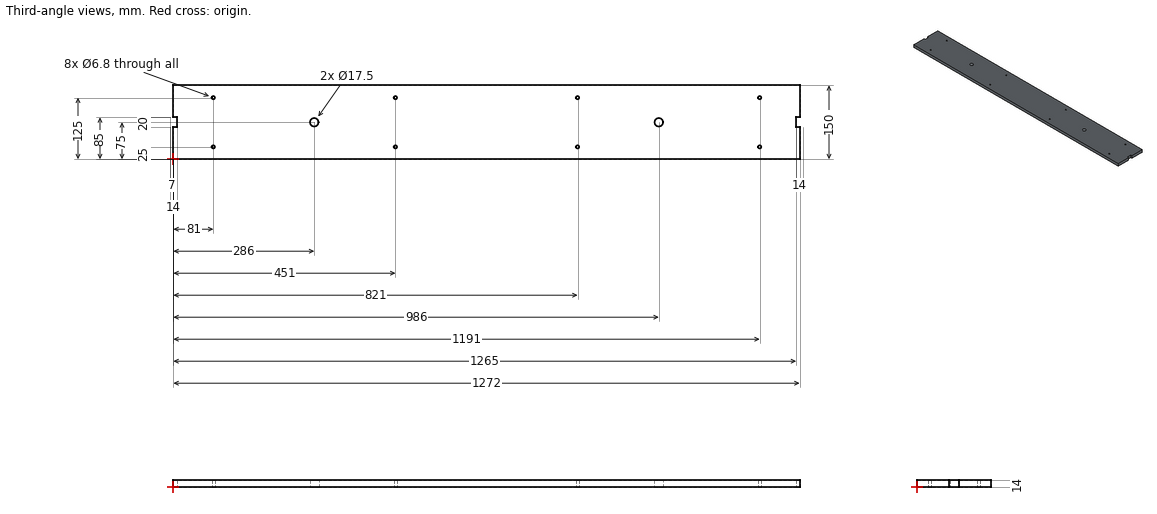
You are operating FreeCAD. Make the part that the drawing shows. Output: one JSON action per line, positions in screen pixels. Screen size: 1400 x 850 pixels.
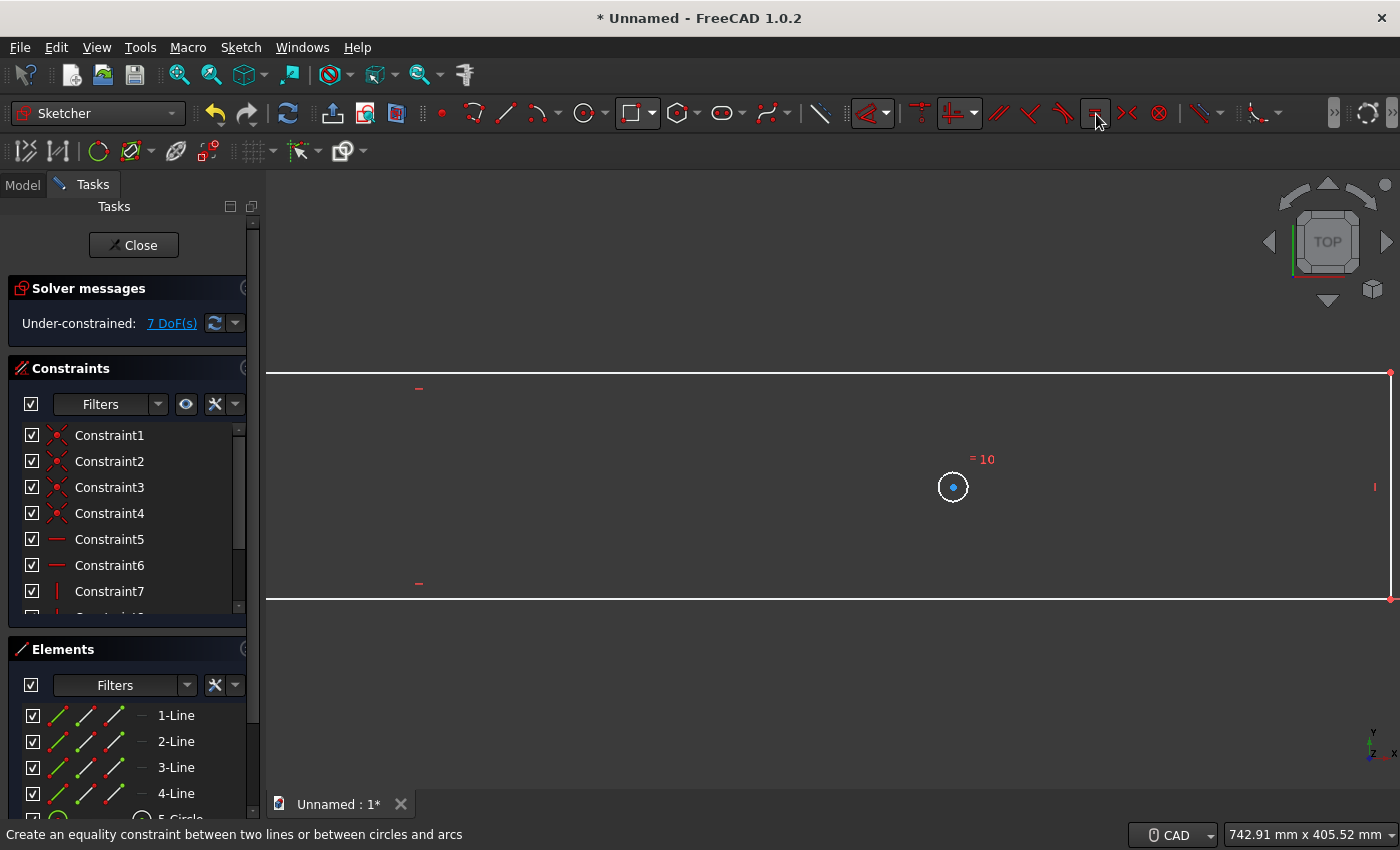
{"action": "scroll", "coordinate": [965, 476], "scroll_direction": "down", "scroll_amount": 5}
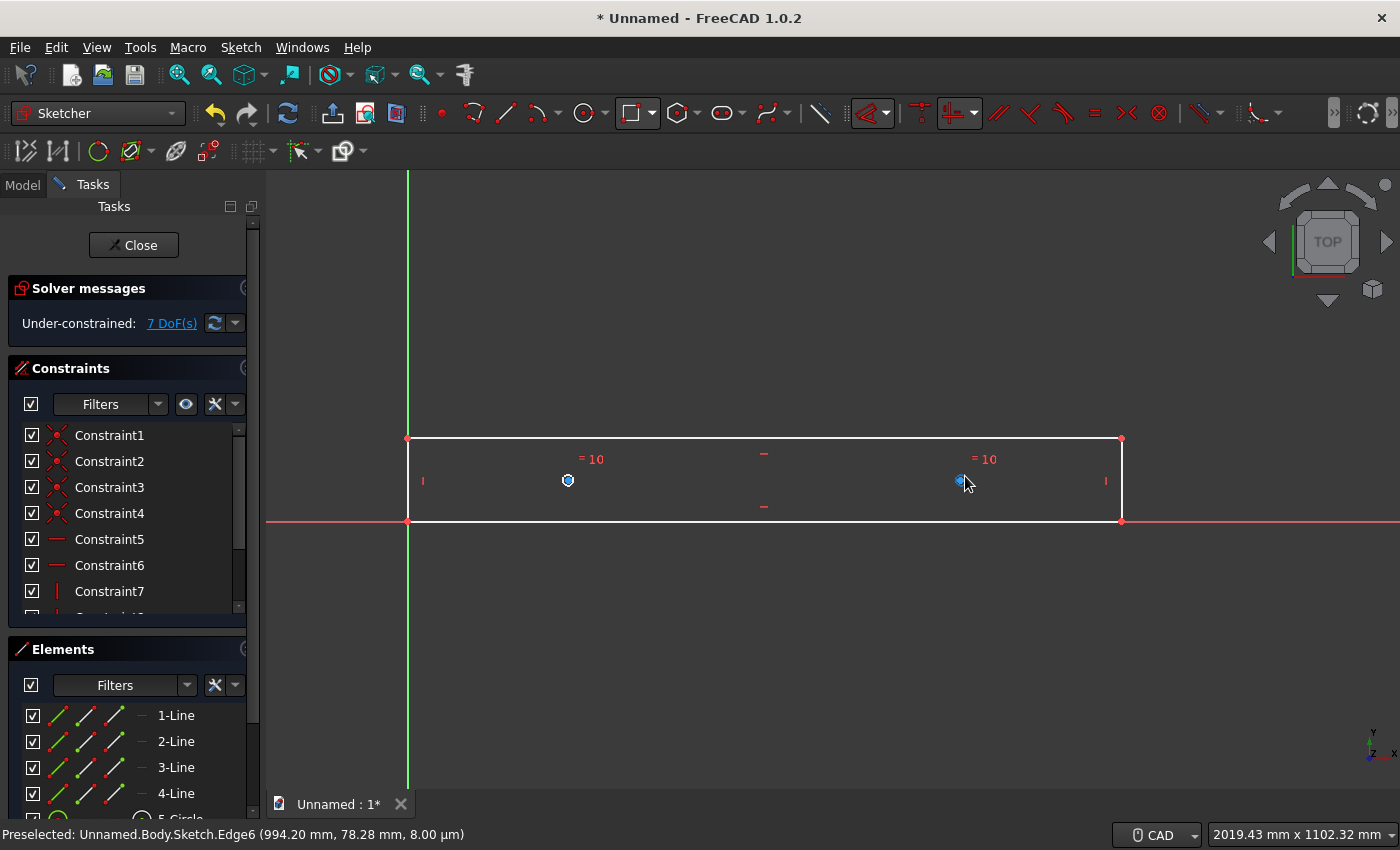
{"action": "left_click", "coordinate": [568, 480]}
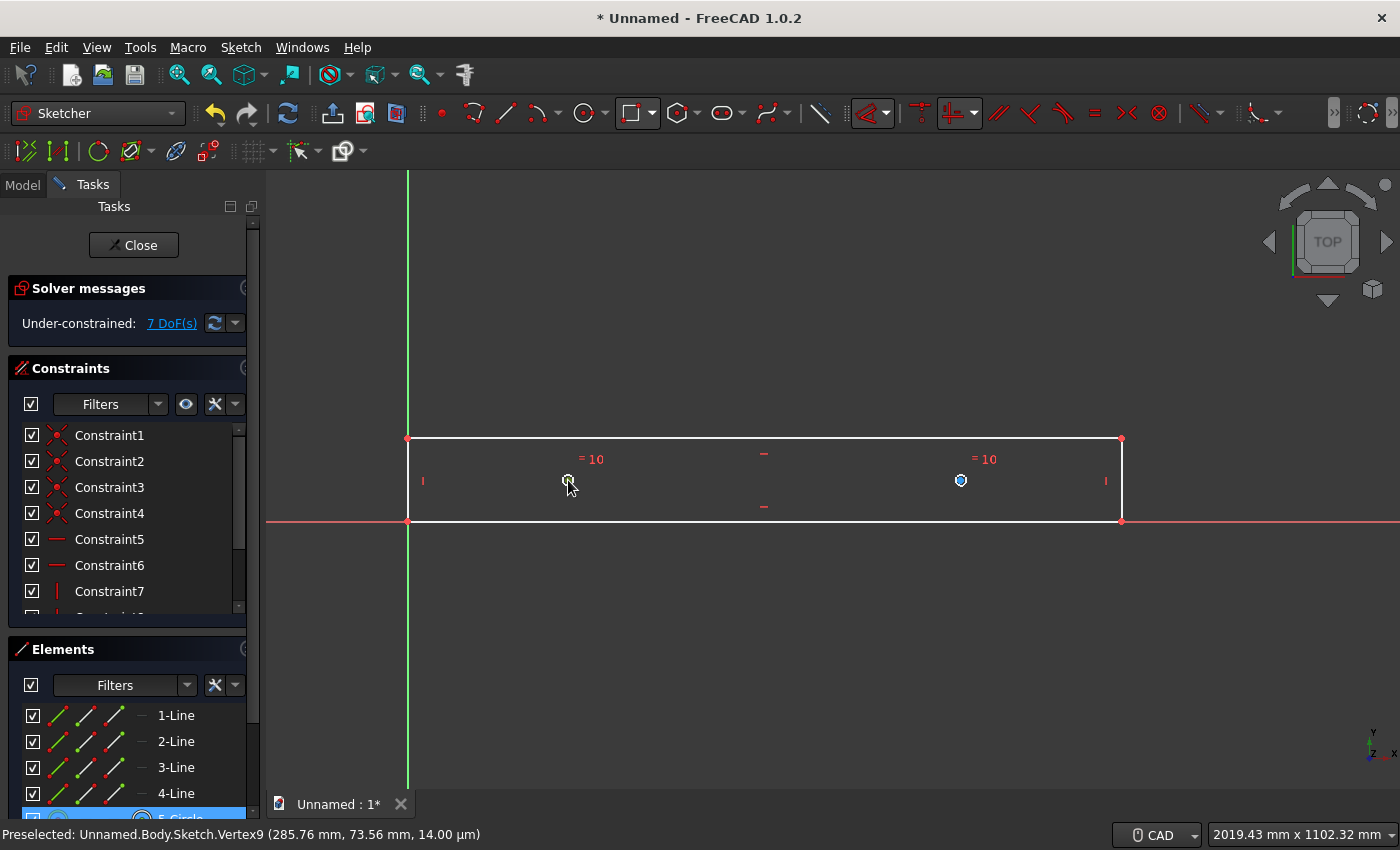
{"action": "left_click", "coordinate": [961, 480]}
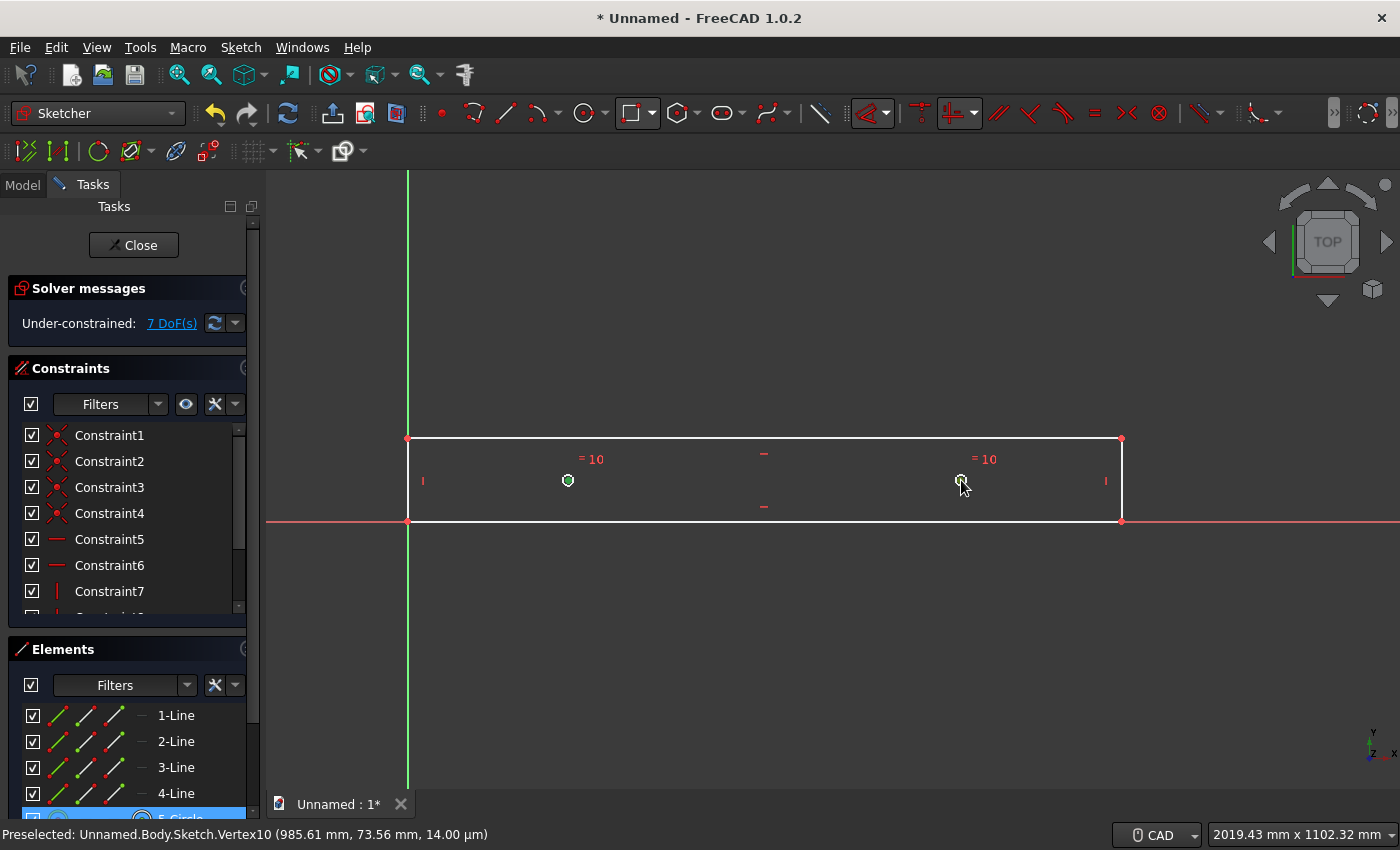
{"action": "left_click", "coordinate": [976, 114]}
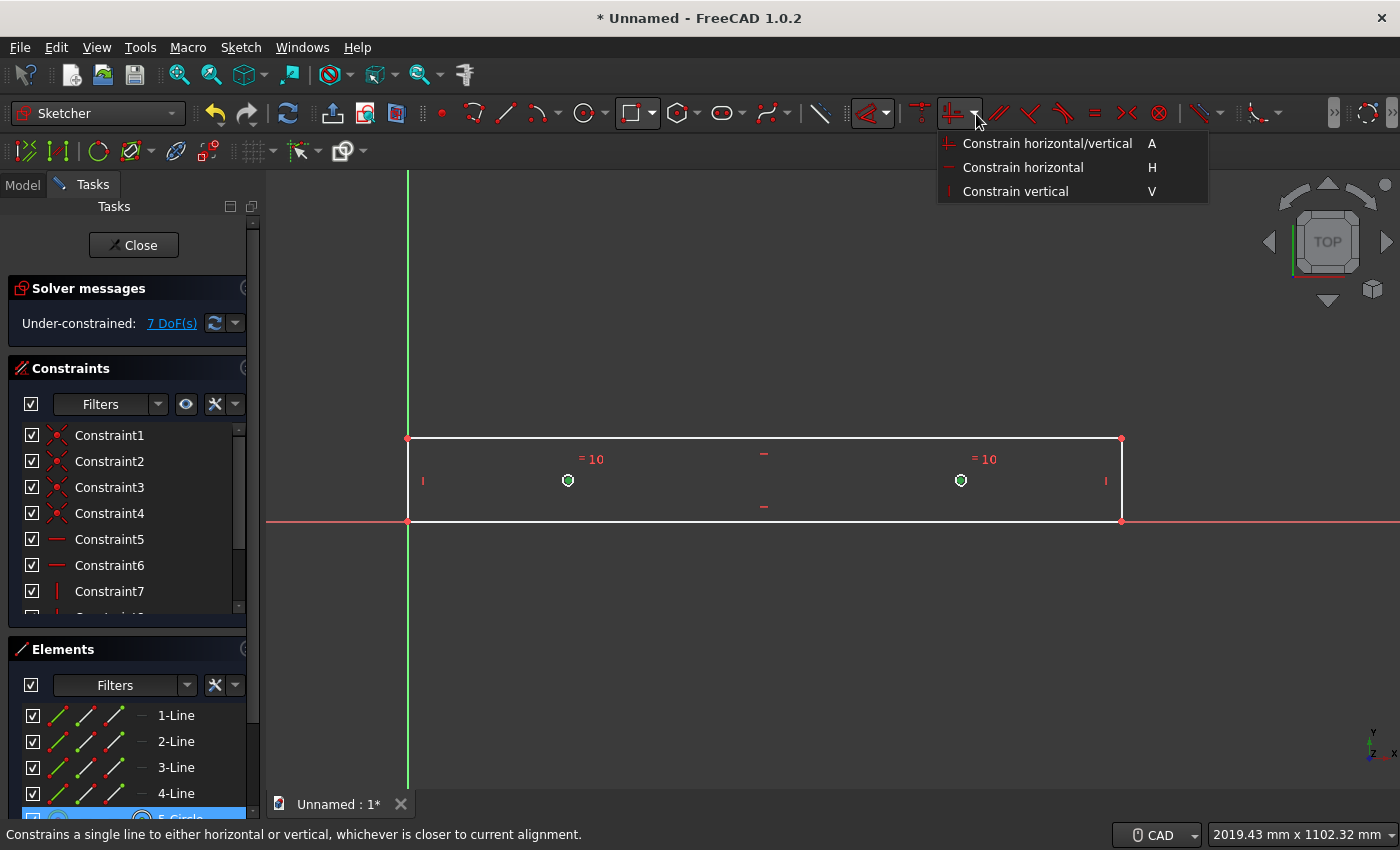
{"action": "left_click", "coordinate": [1073, 167]}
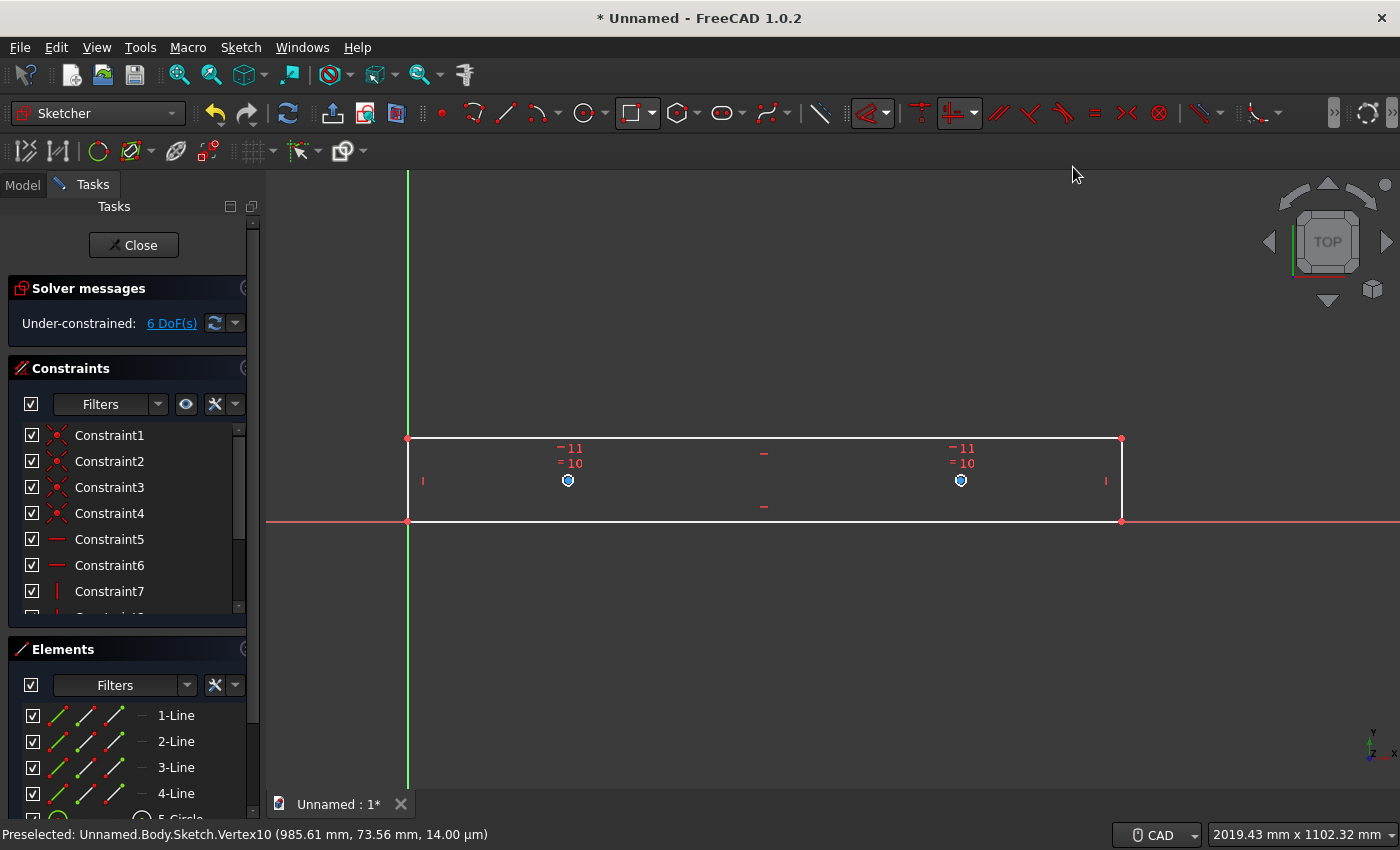
{"action": "scroll", "coordinate": [563, 480], "scroll_direction": "up", "scroll_amount": 7}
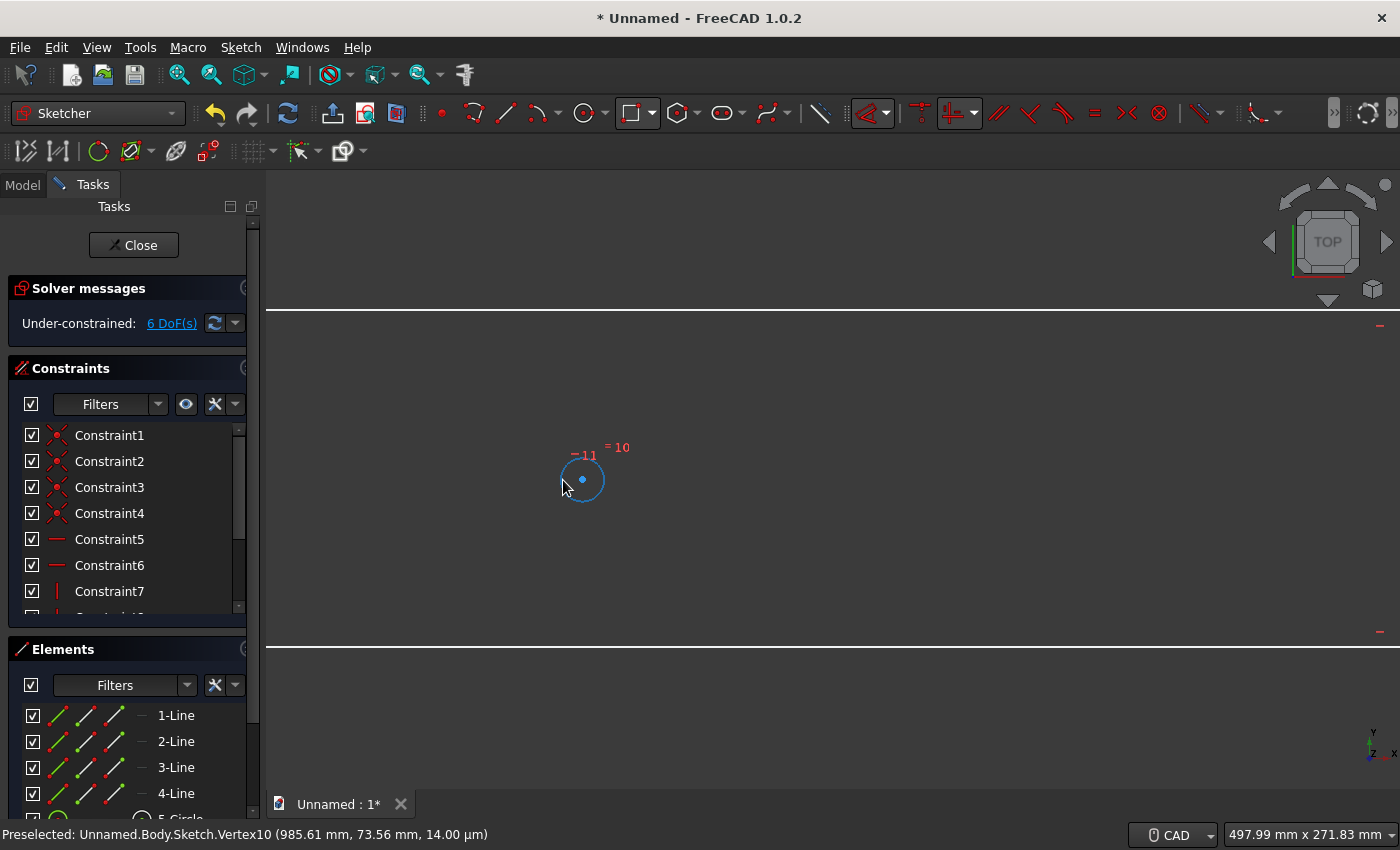
{"action": "left_click", "coordinate": [561, 479]}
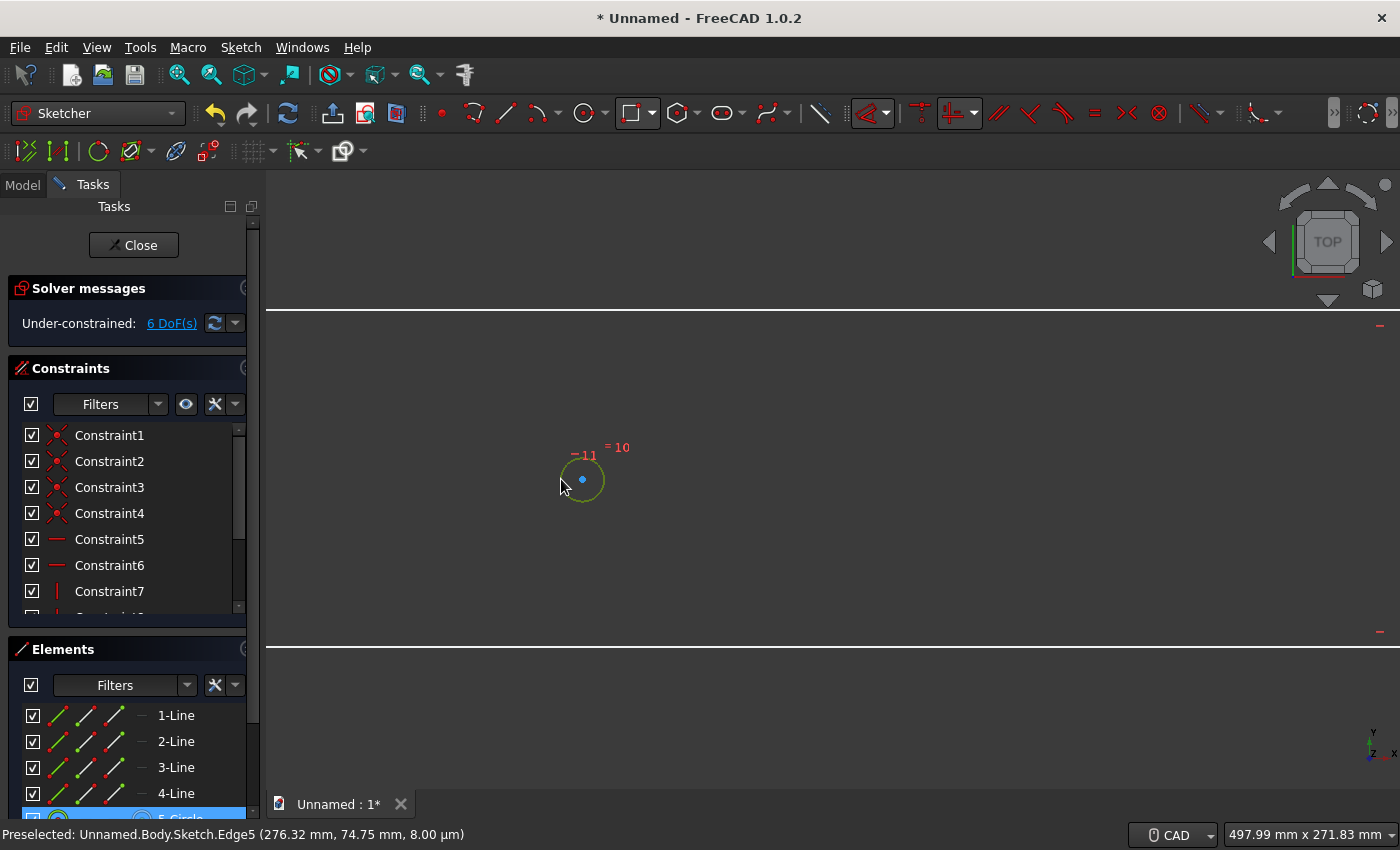
{"action": "left_click", "coordinate": [888, 114]}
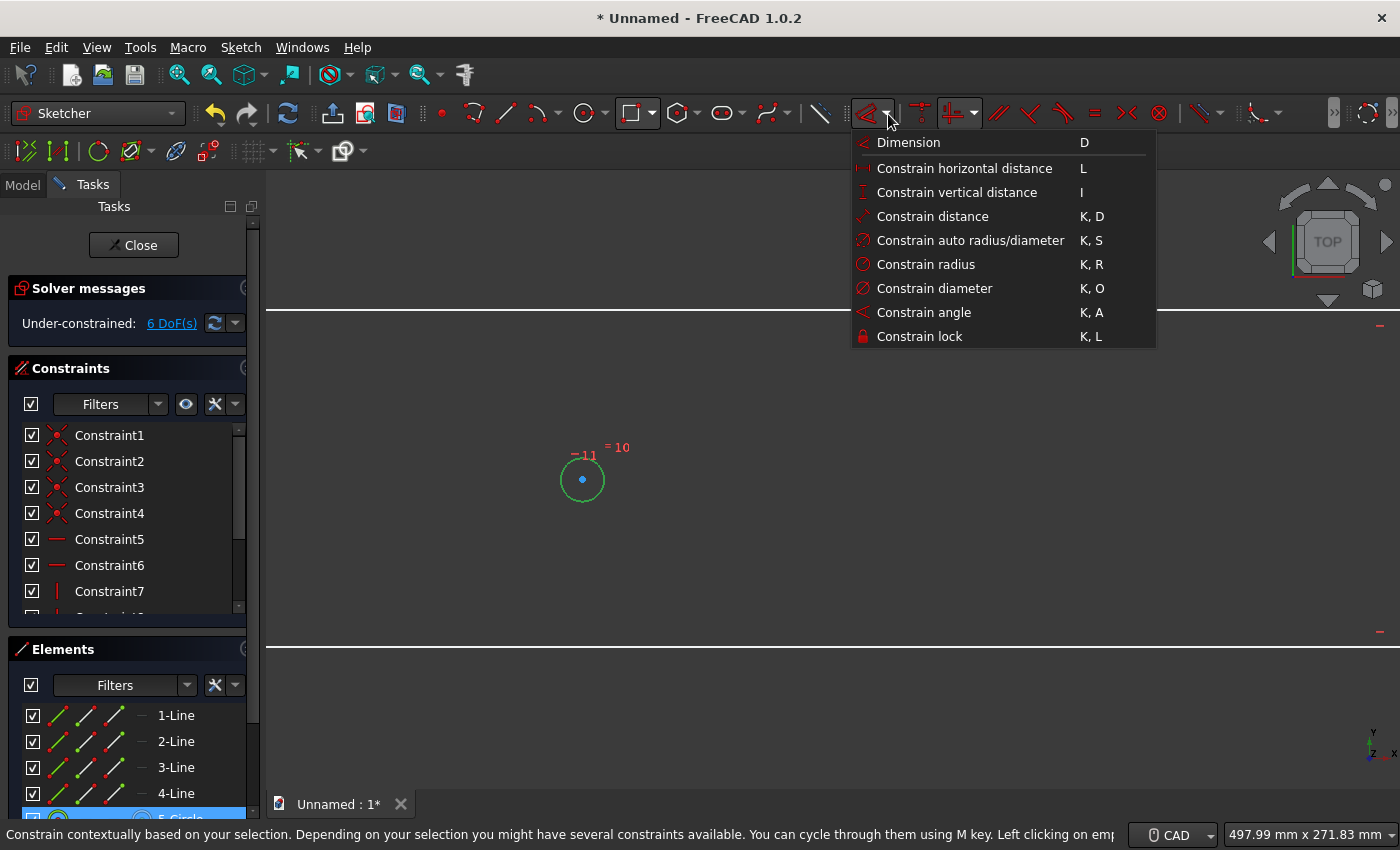
{"action": "left_click", "coordinate": [1004, 288]}